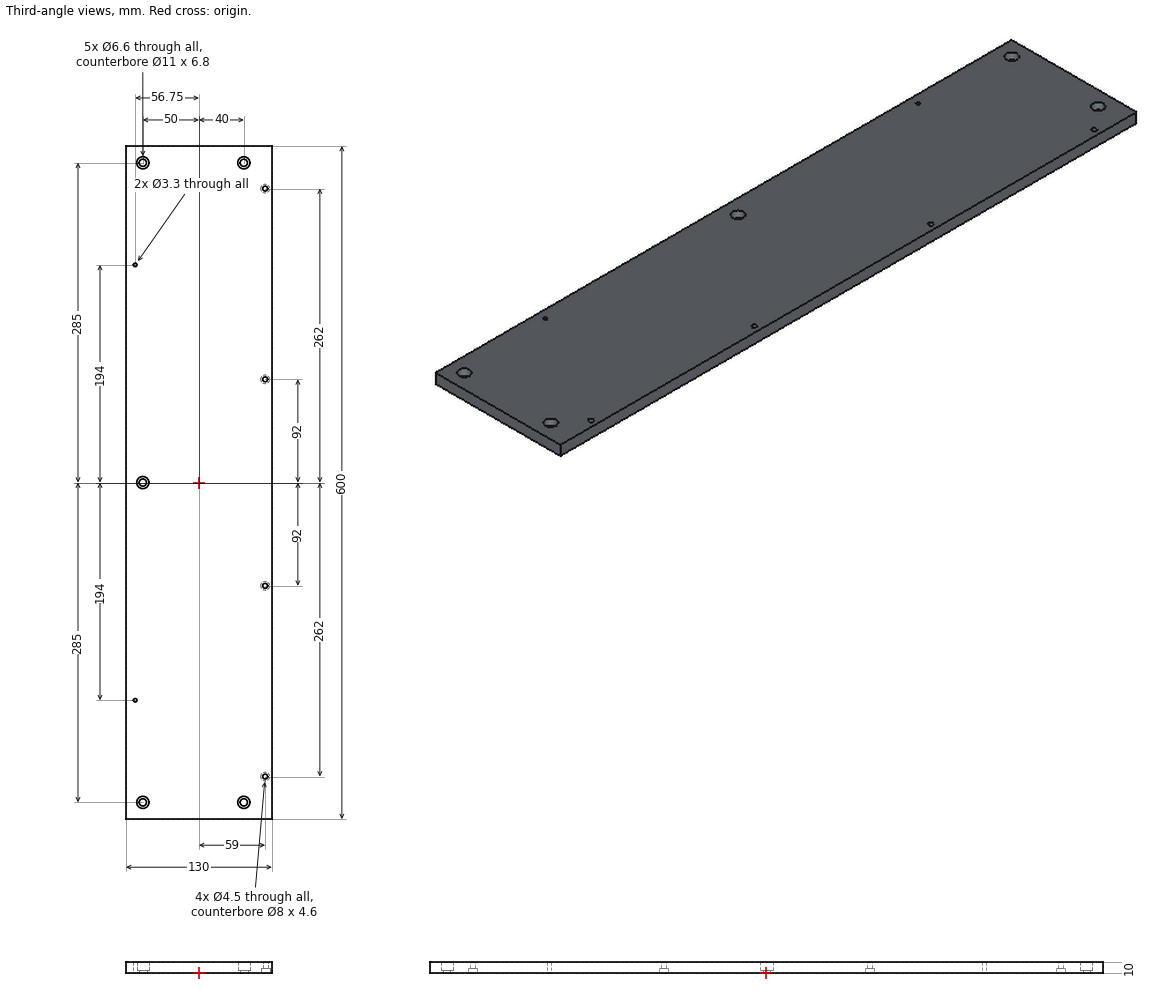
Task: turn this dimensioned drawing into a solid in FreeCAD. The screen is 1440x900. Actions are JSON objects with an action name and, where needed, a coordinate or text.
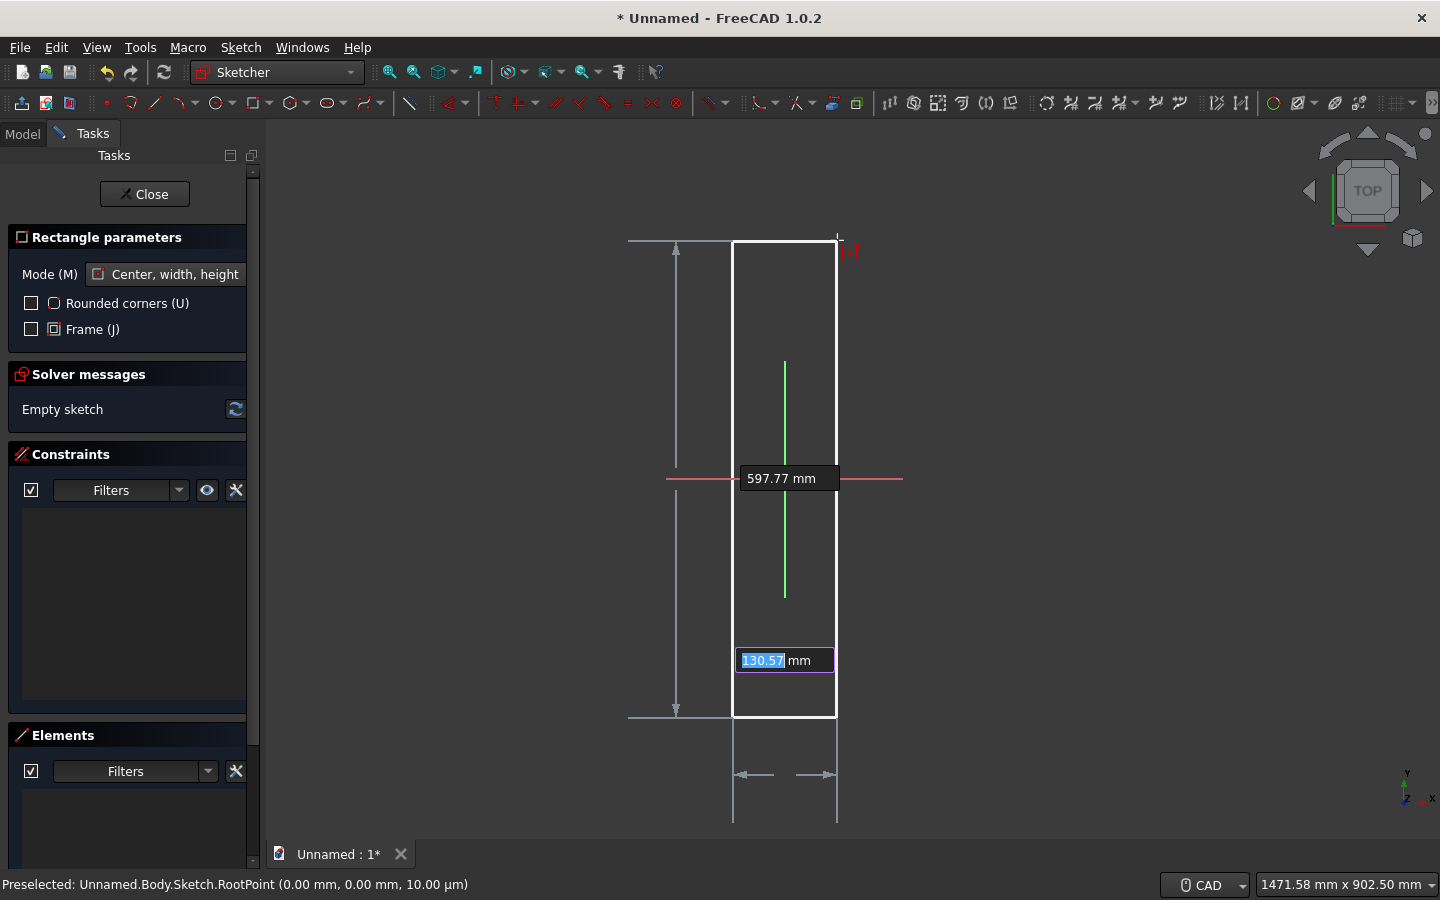
{"action": "type", "text": "130"}
{"action": "key", "text": "Tab"}
{"action": "type", "text": "600"}
{"action": "key", "text": "Return"}
{"action": "key", "text": "Escape"}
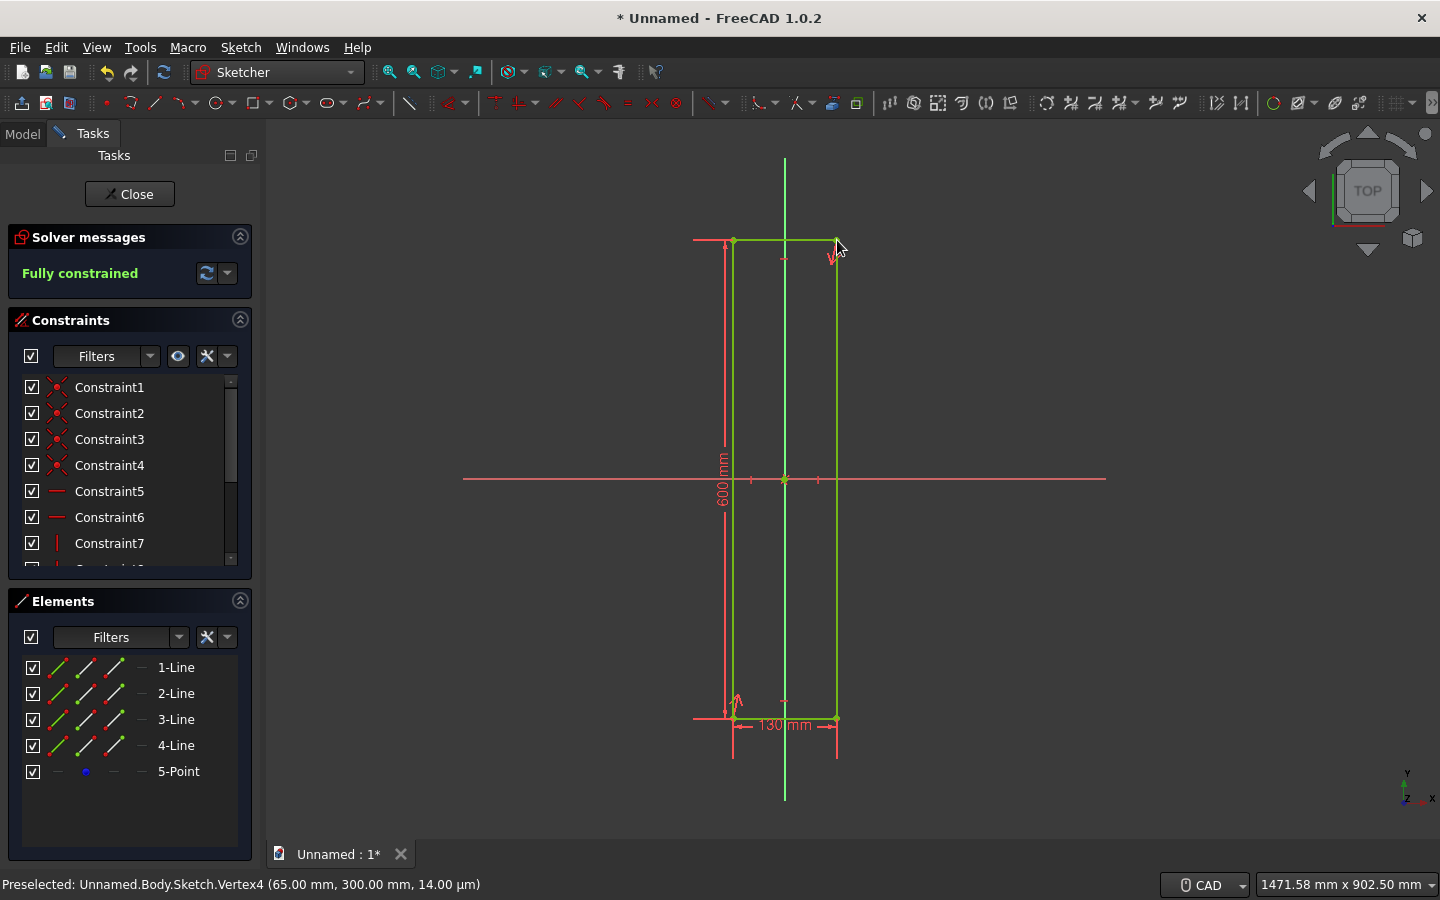
{"action": "left_click", "coordinate": [130, 194]}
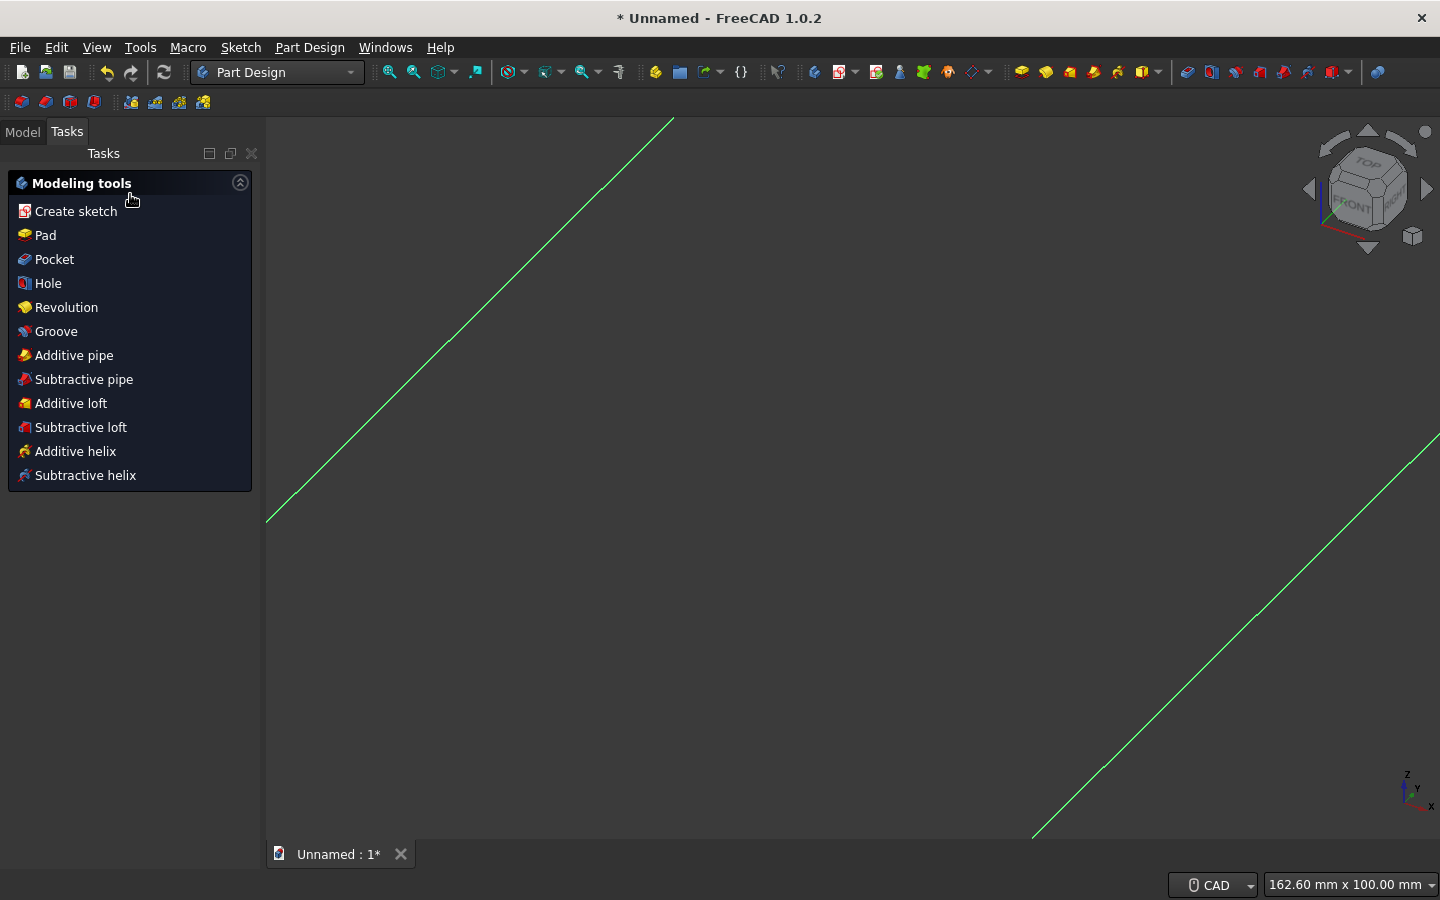
{"action": "left_click", "coordinate": [1022, 72]}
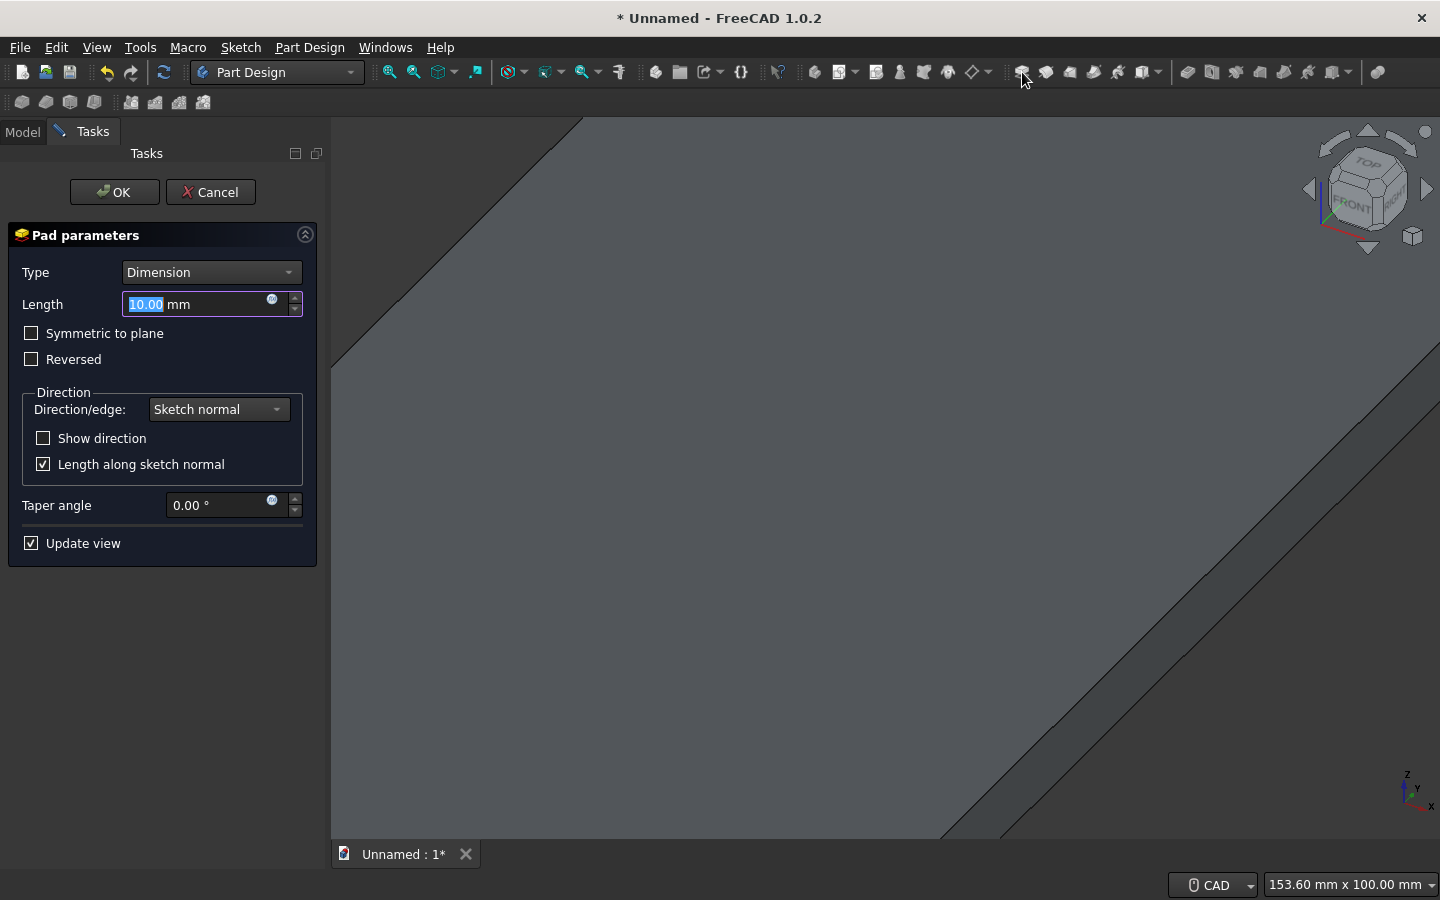
{"action": "type", "text": "10"}
{"action": "key", "text": "Tab"}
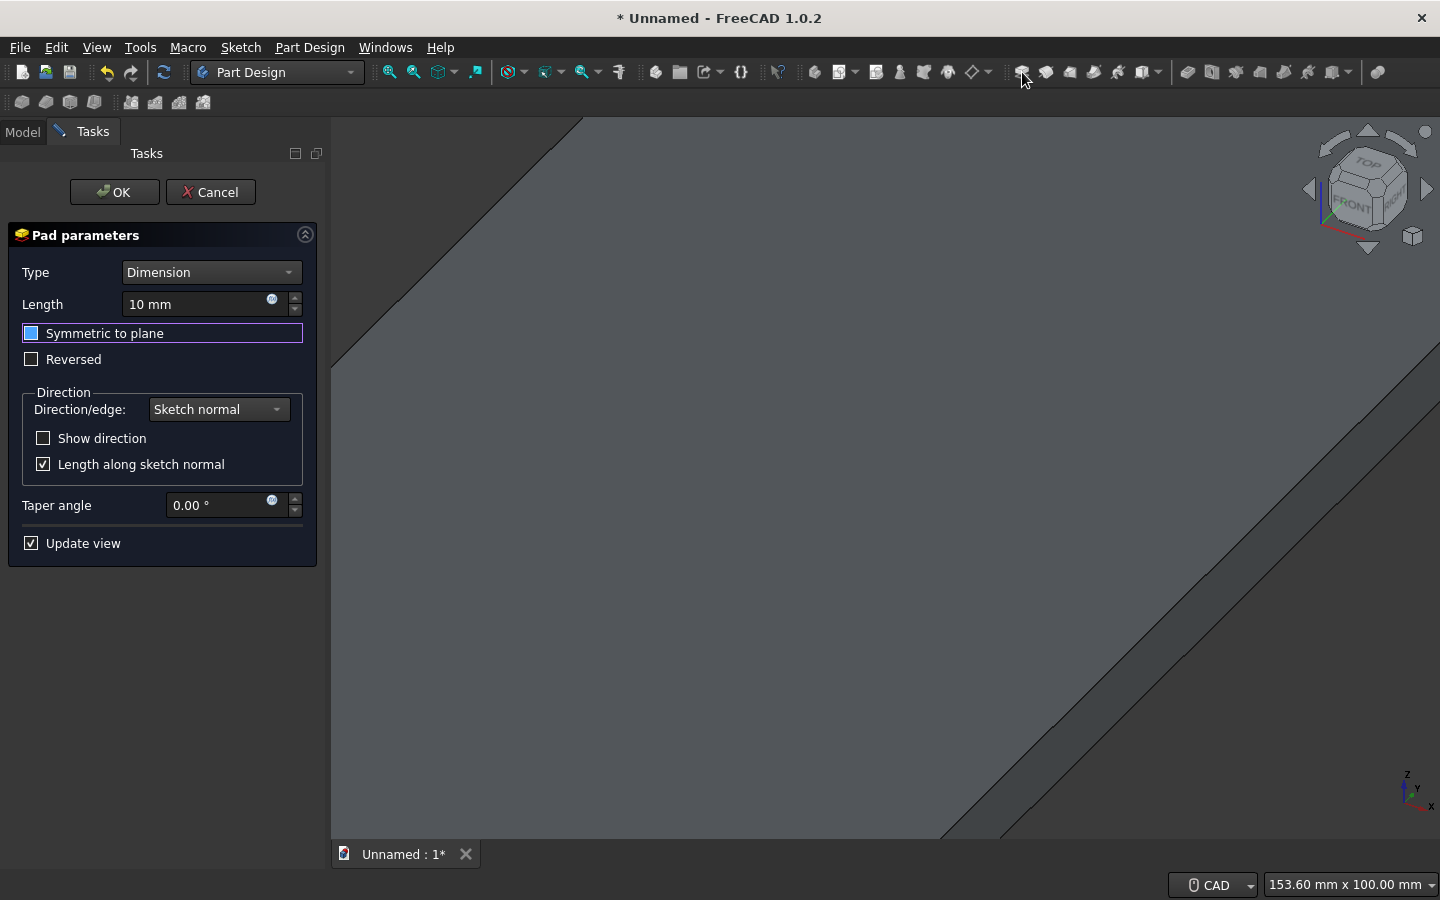
{"action": "left_click", "coordinate": [115, 192]}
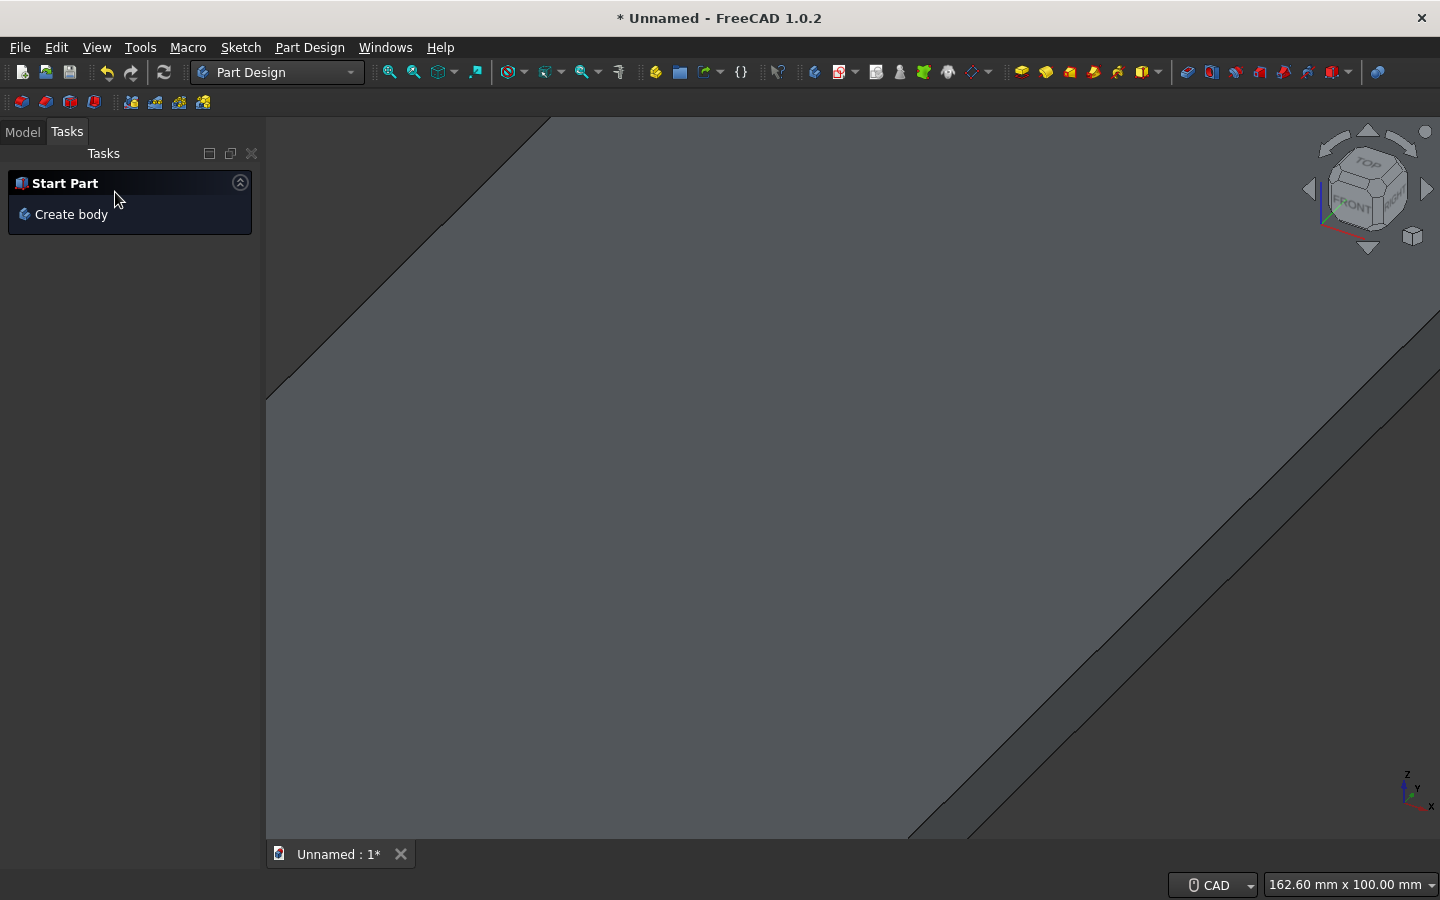
{"action": "key", "text": "v f"}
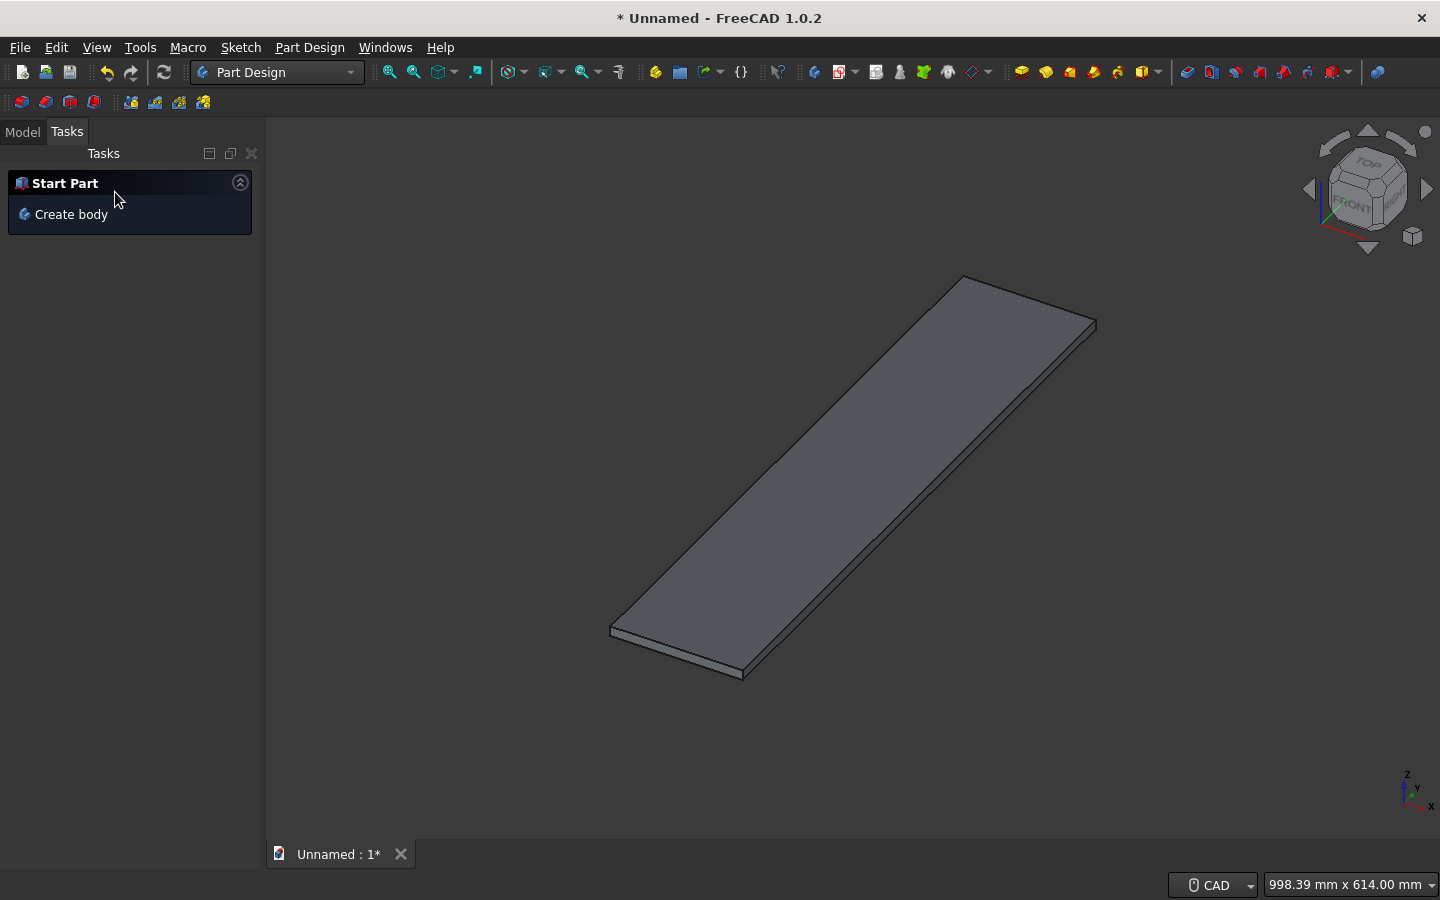
{"action": "left_click", "coordinate": [954, 372]}